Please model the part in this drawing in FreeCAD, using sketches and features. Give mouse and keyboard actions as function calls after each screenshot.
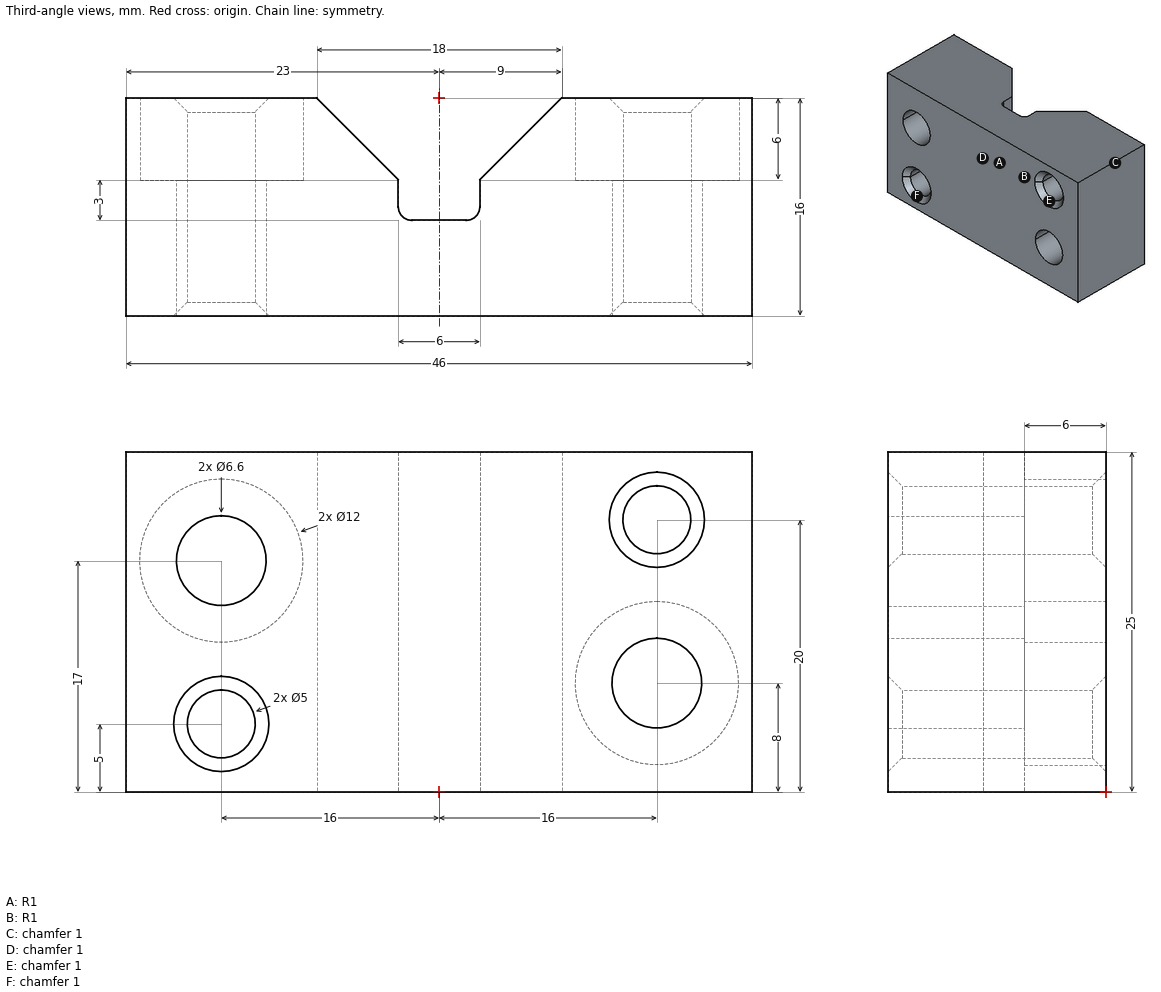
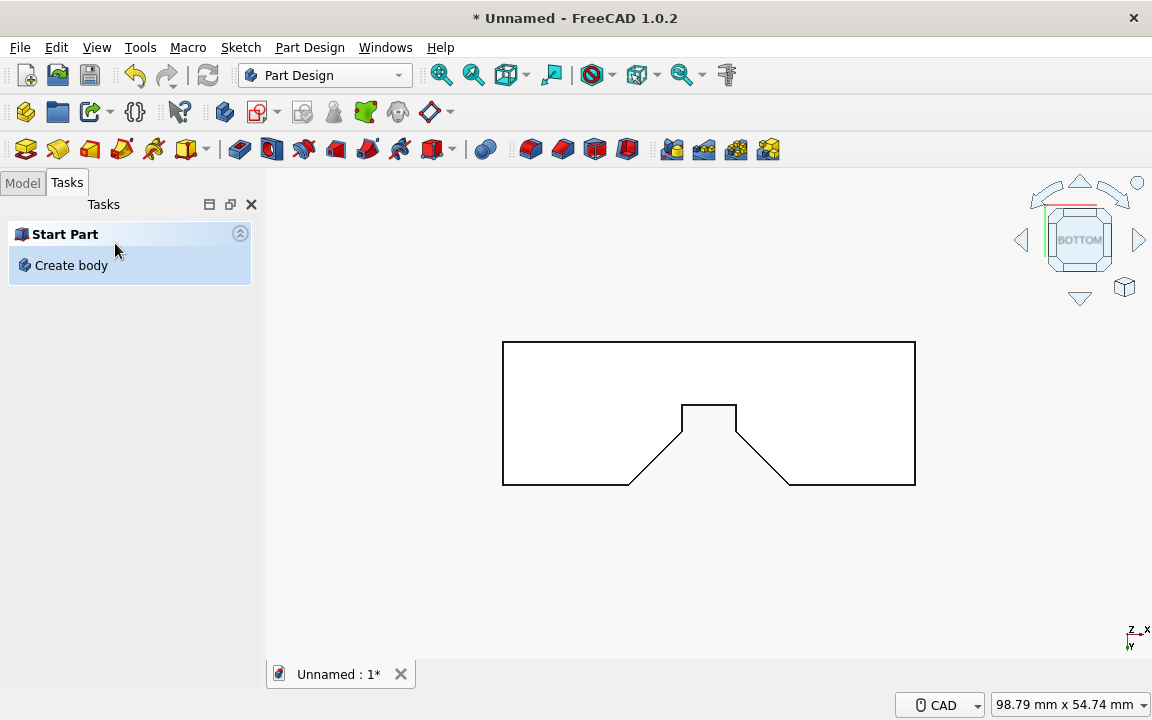
key(4)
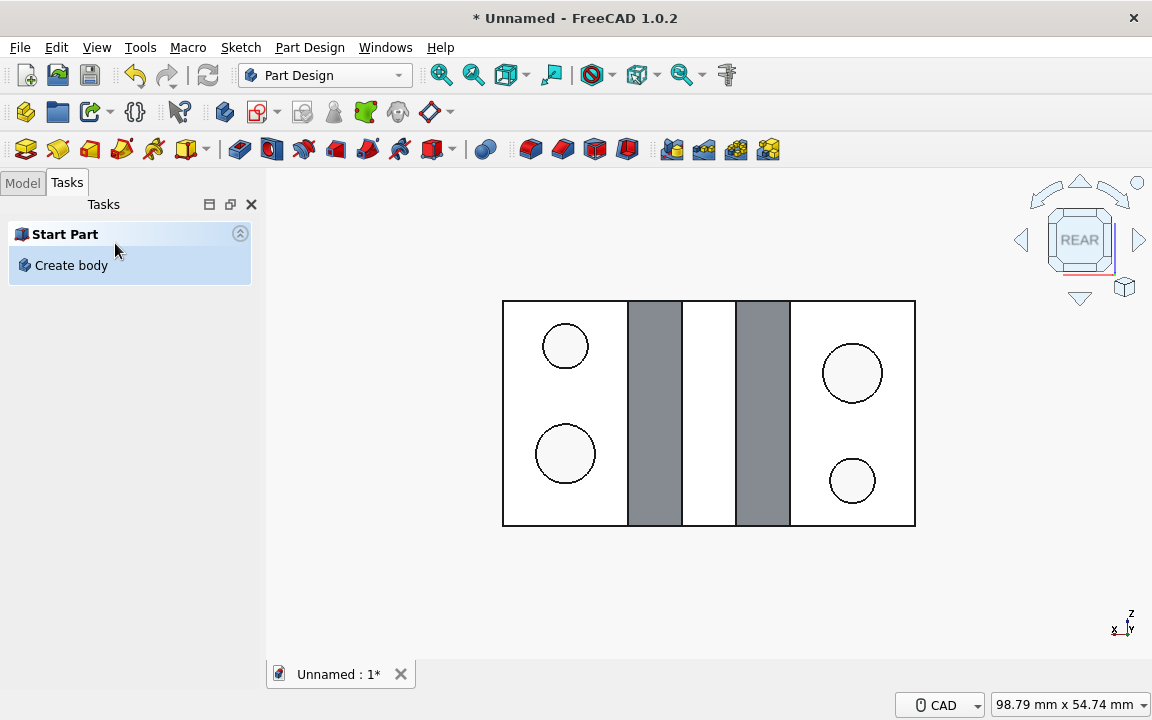
key(6)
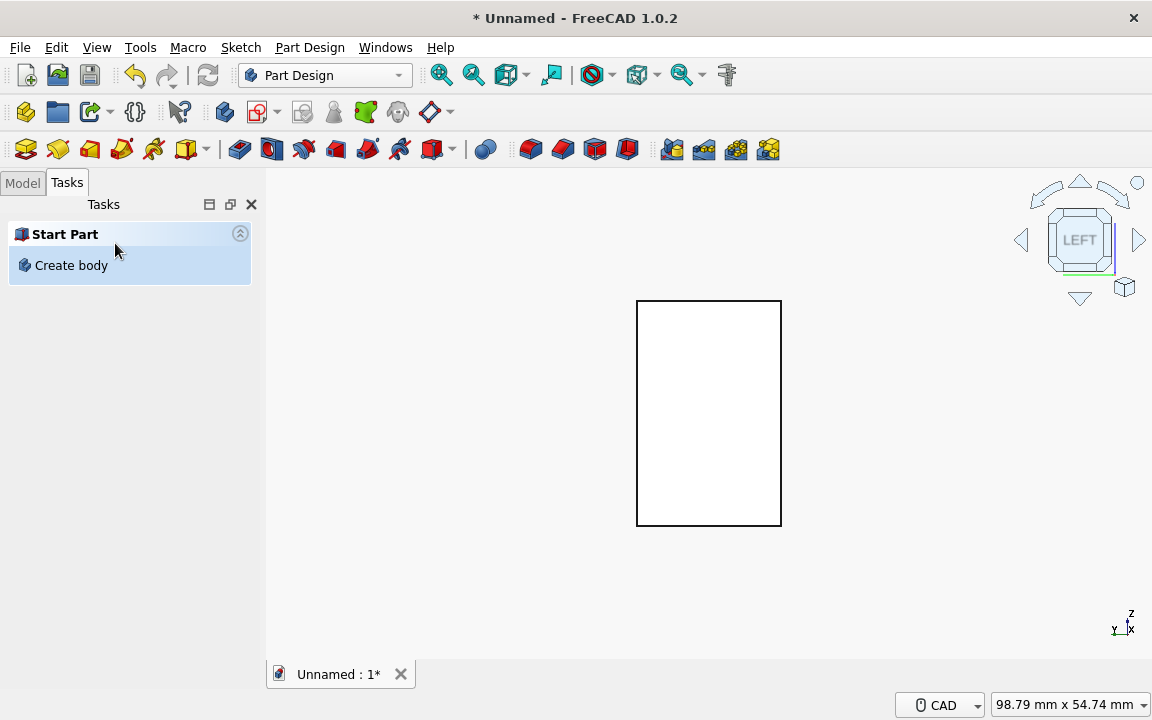
key(v)
key(3)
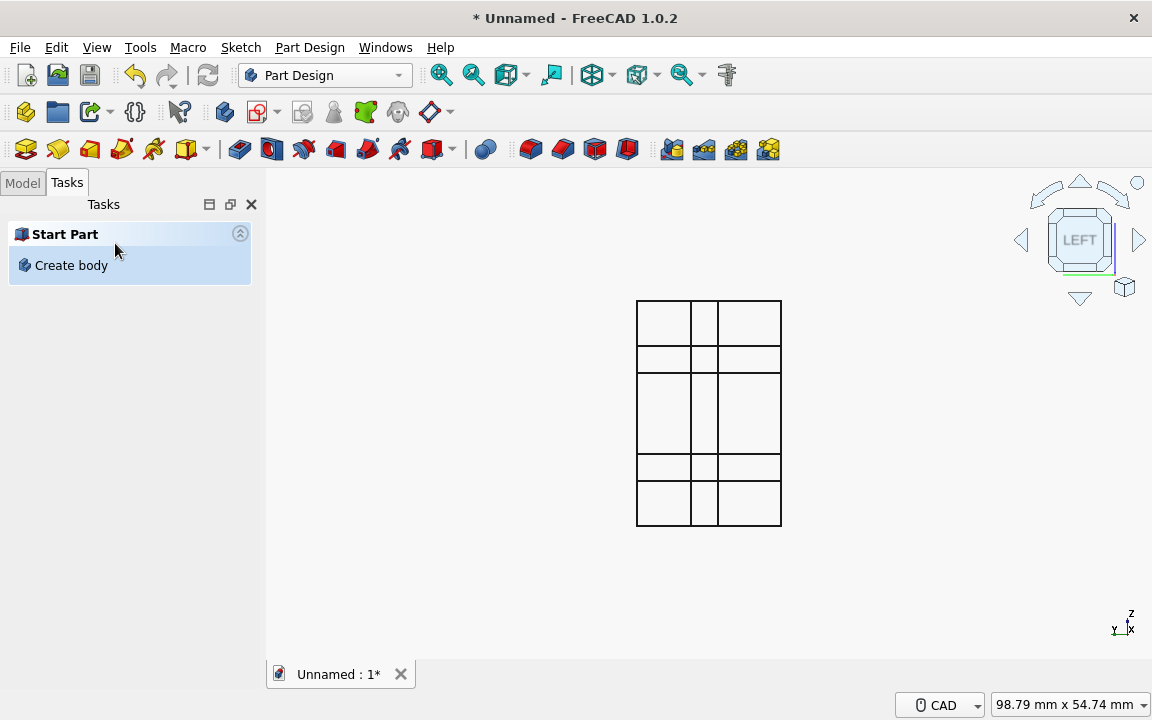
key(0)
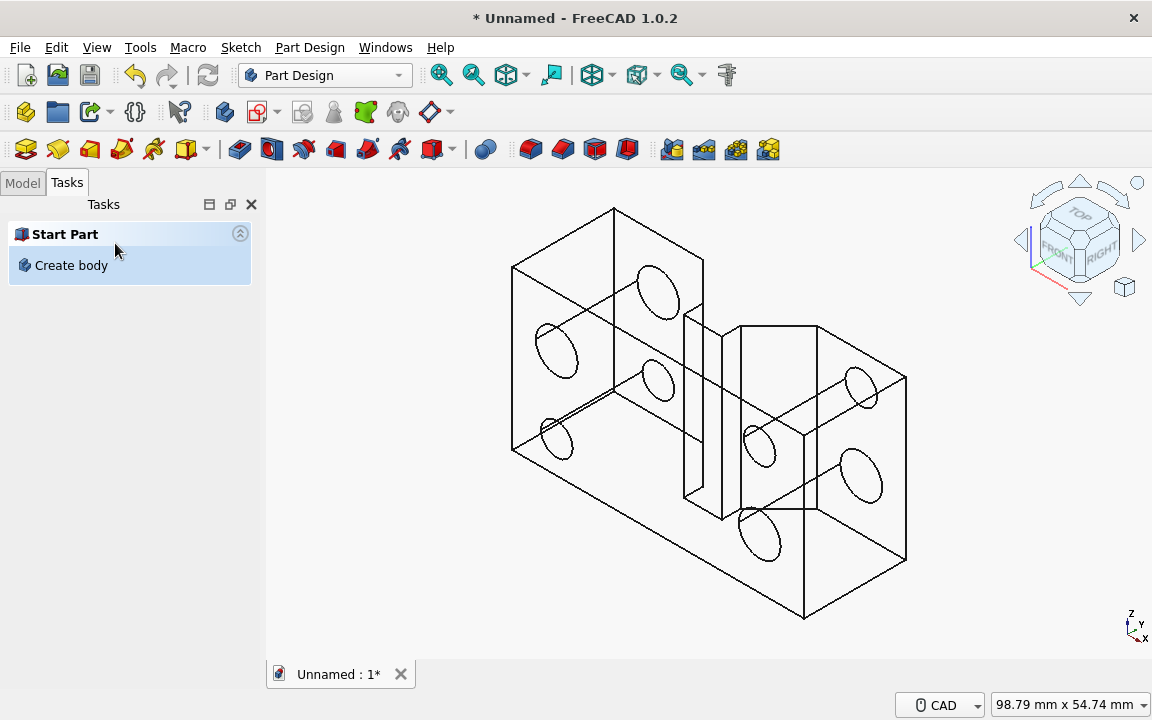
click(684, 405)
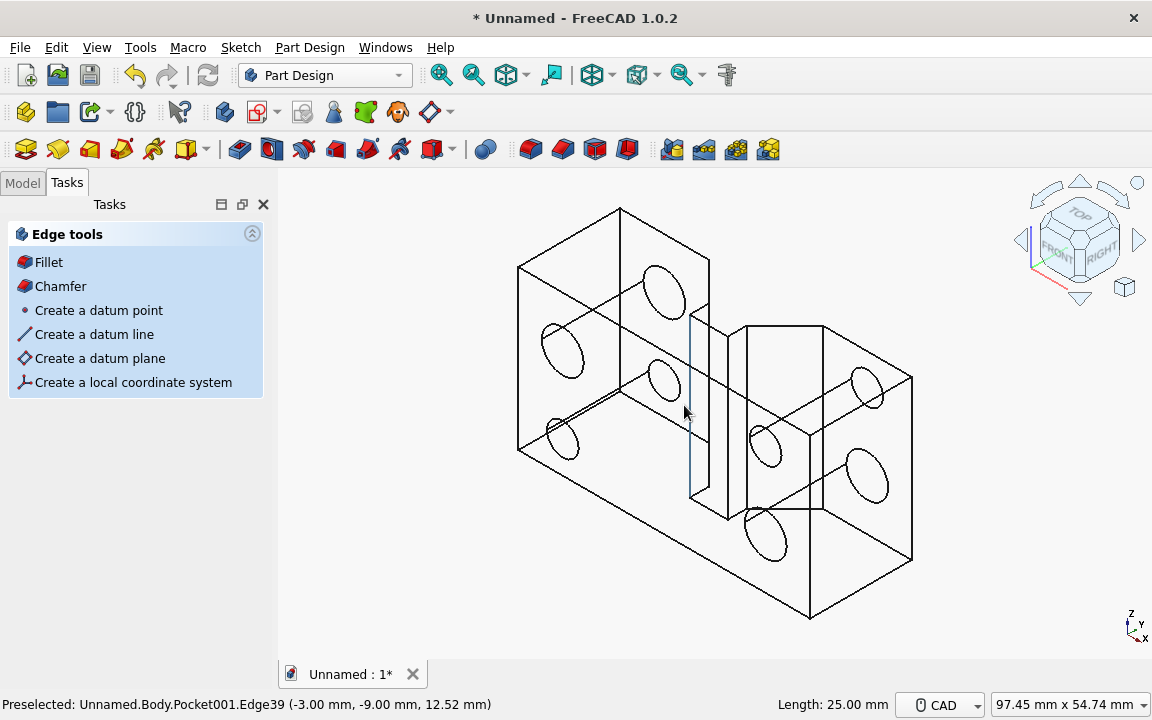
key(v)
key(1)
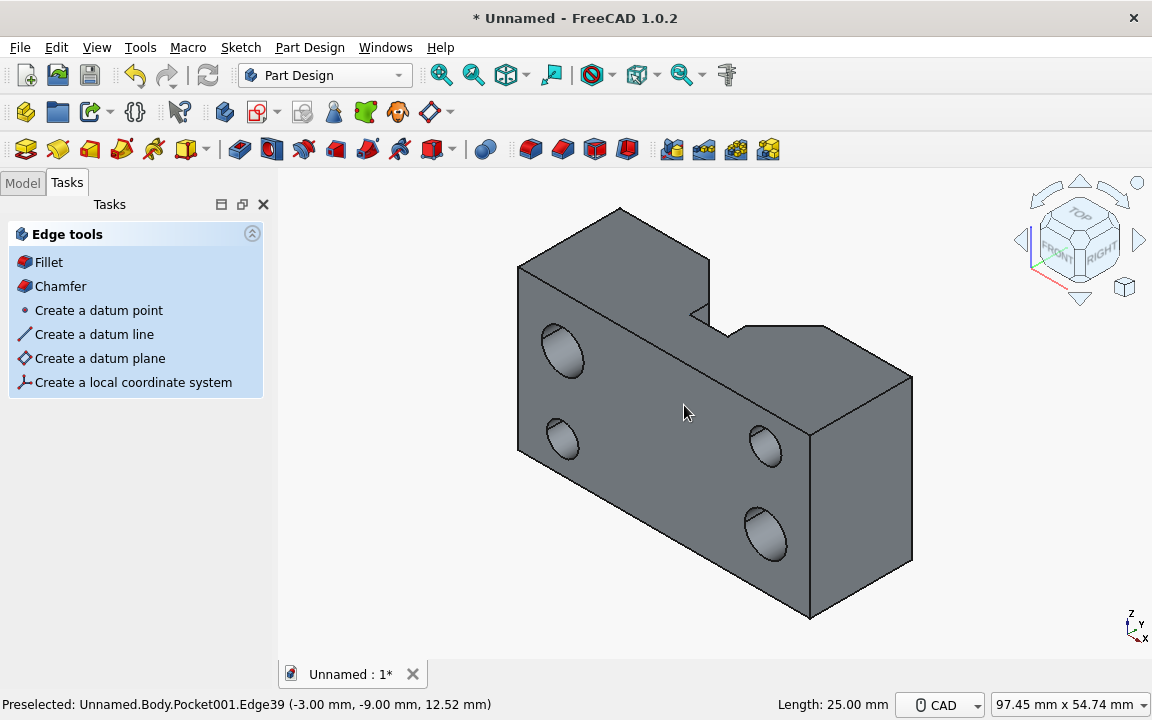
click(532, 150)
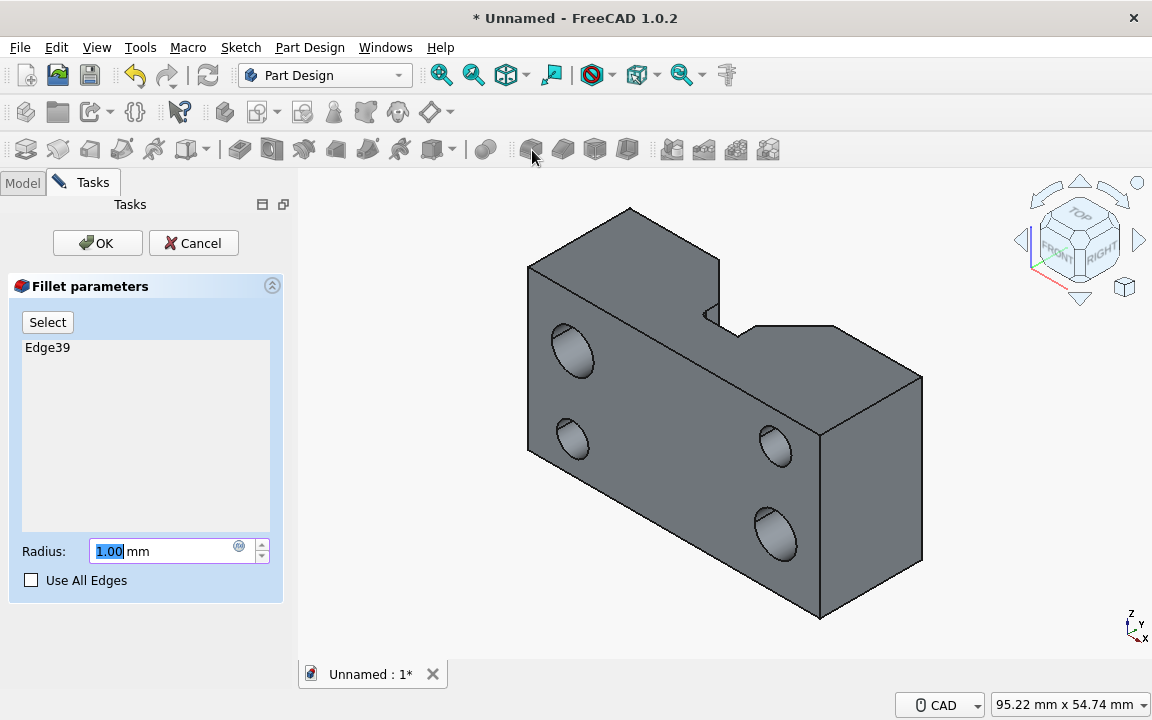
text(1)
key(Tab)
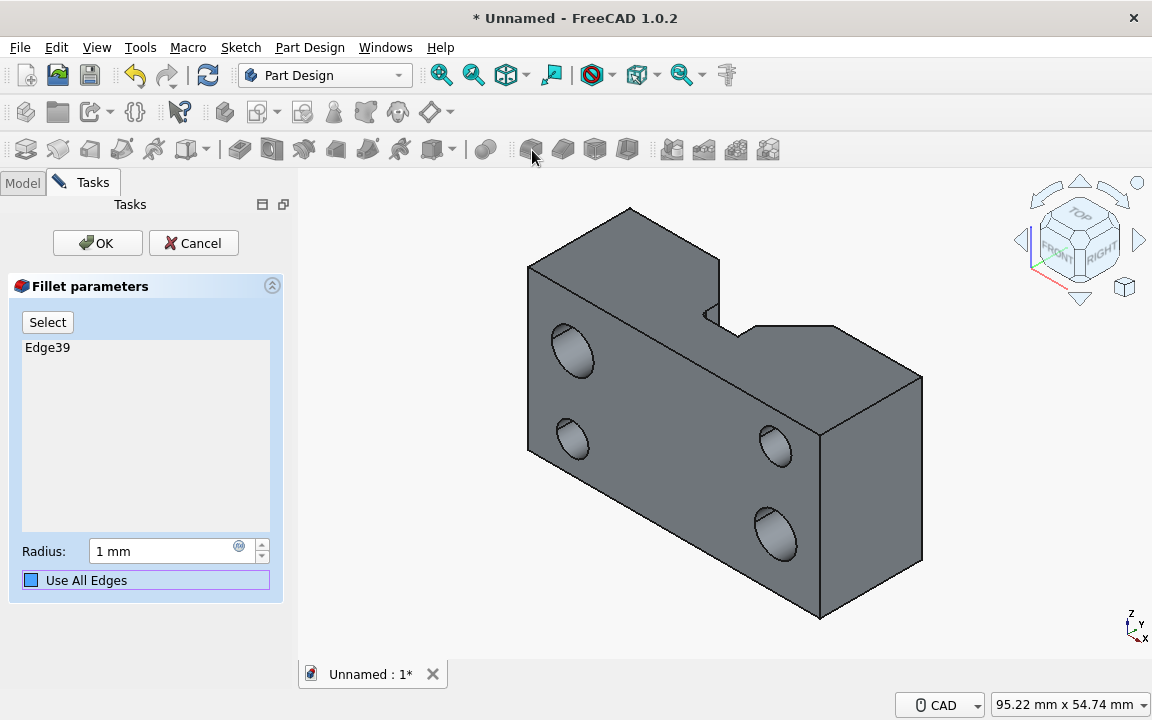
click(98, 243)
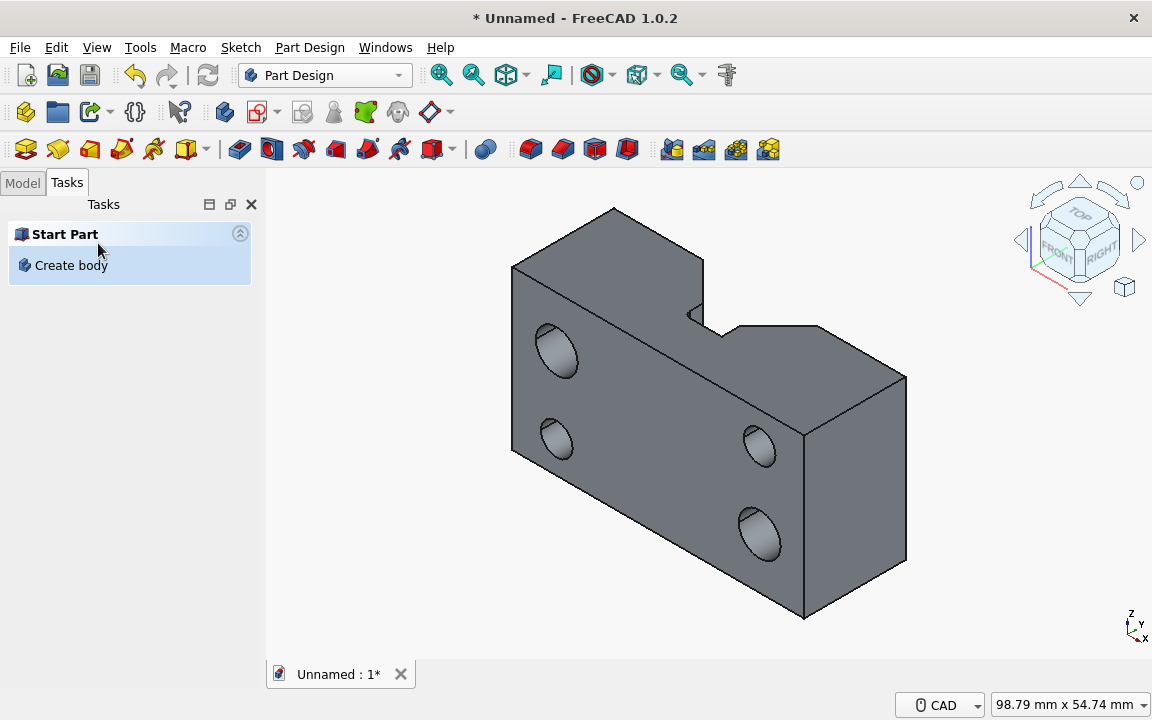
key(2)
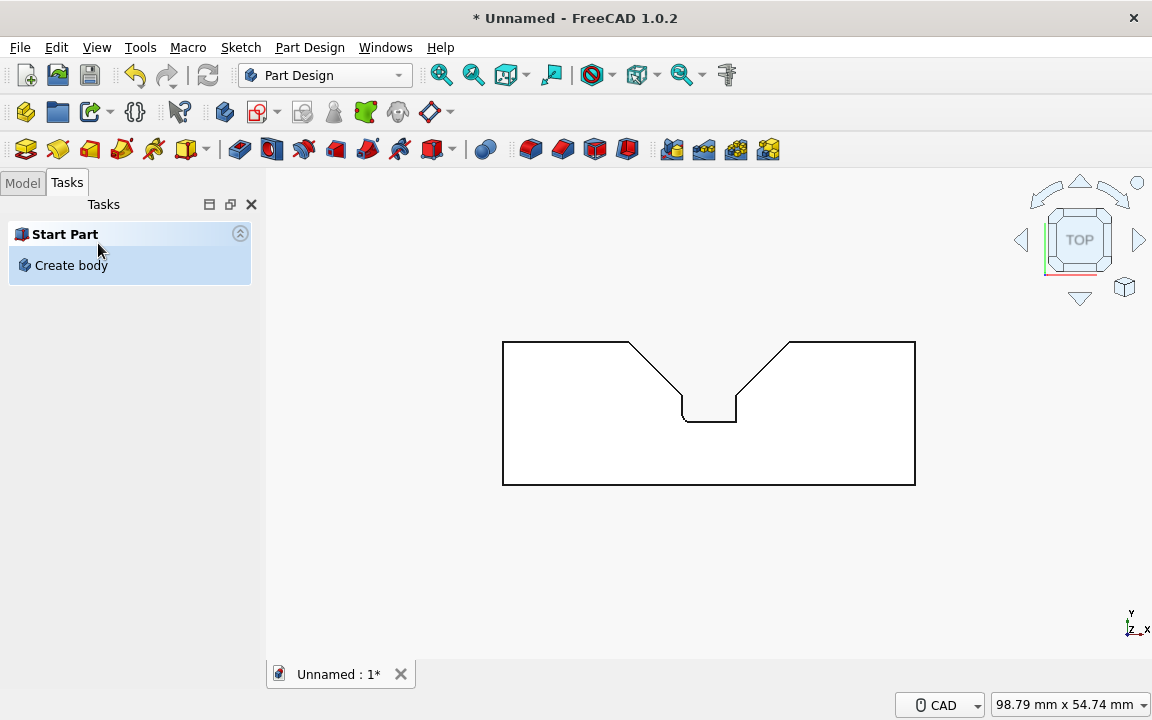
key(0)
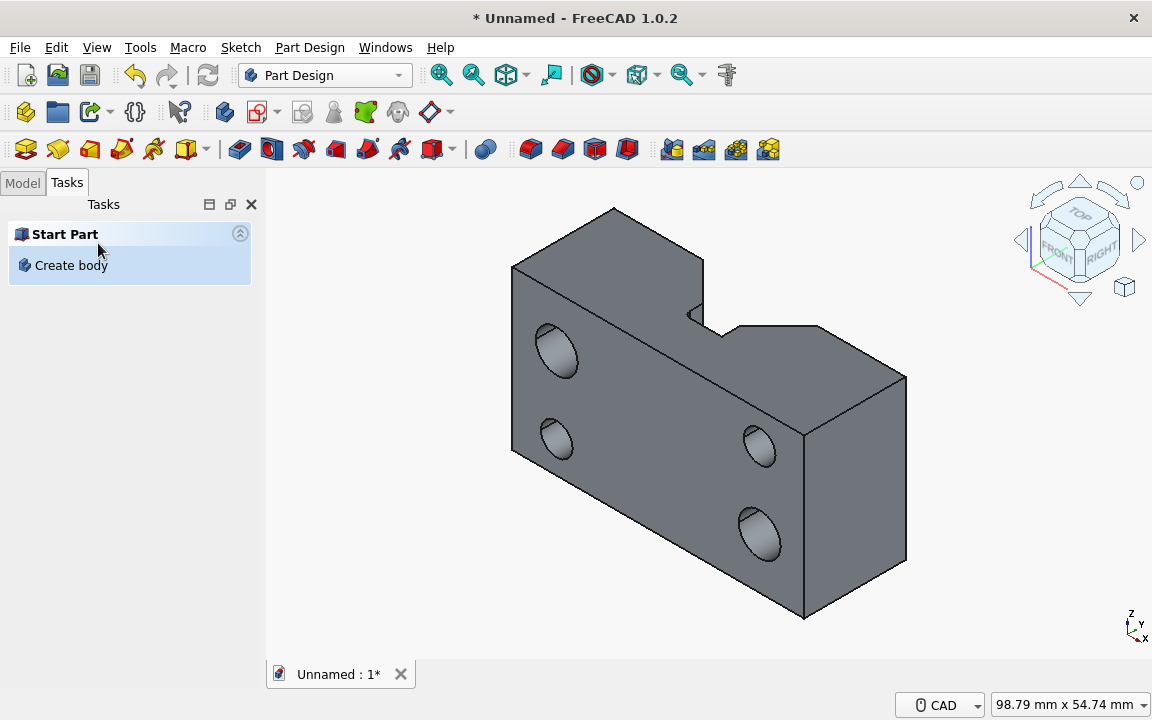
key(1)